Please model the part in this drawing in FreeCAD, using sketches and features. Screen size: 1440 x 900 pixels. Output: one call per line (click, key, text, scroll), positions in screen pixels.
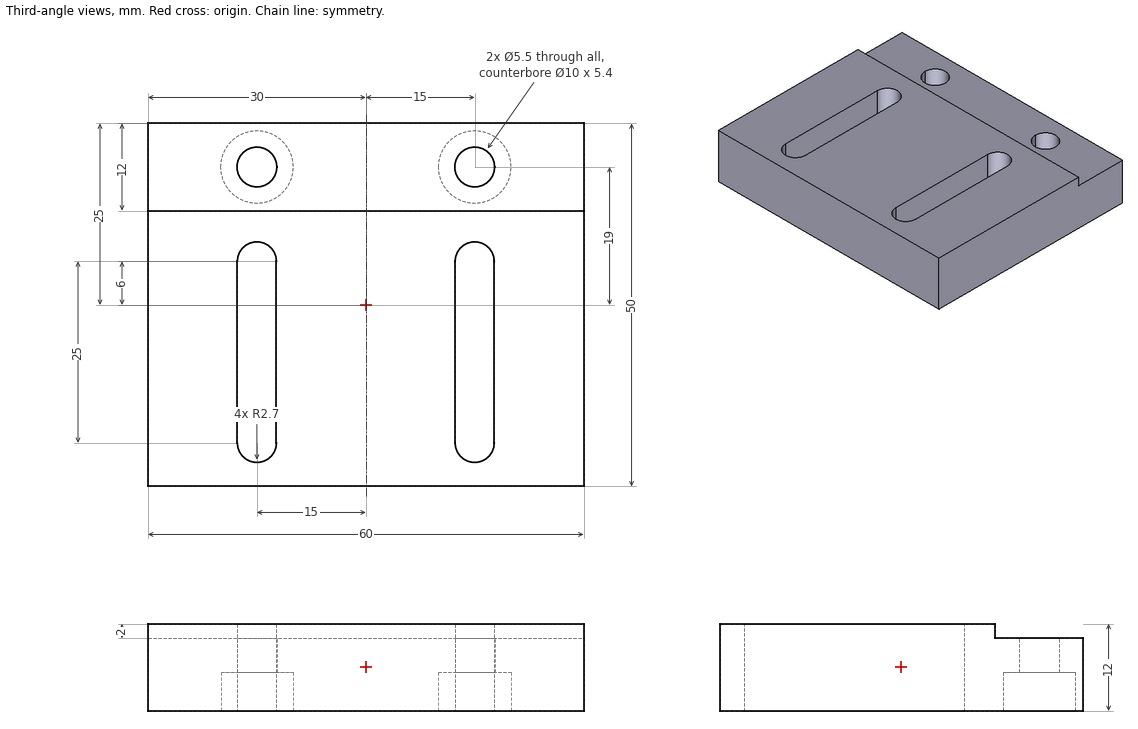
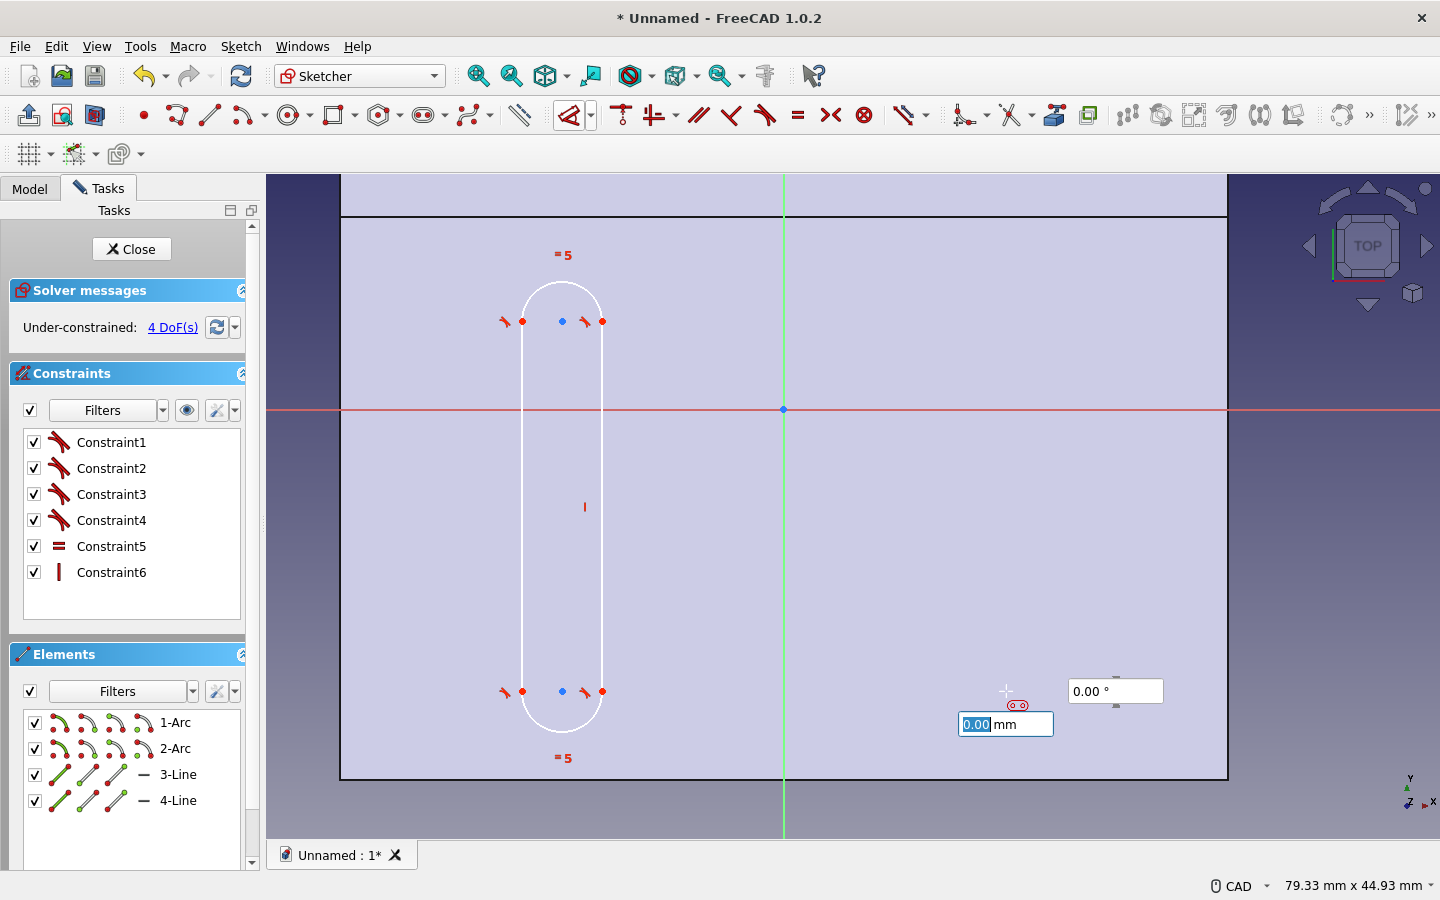
click(1006, 321)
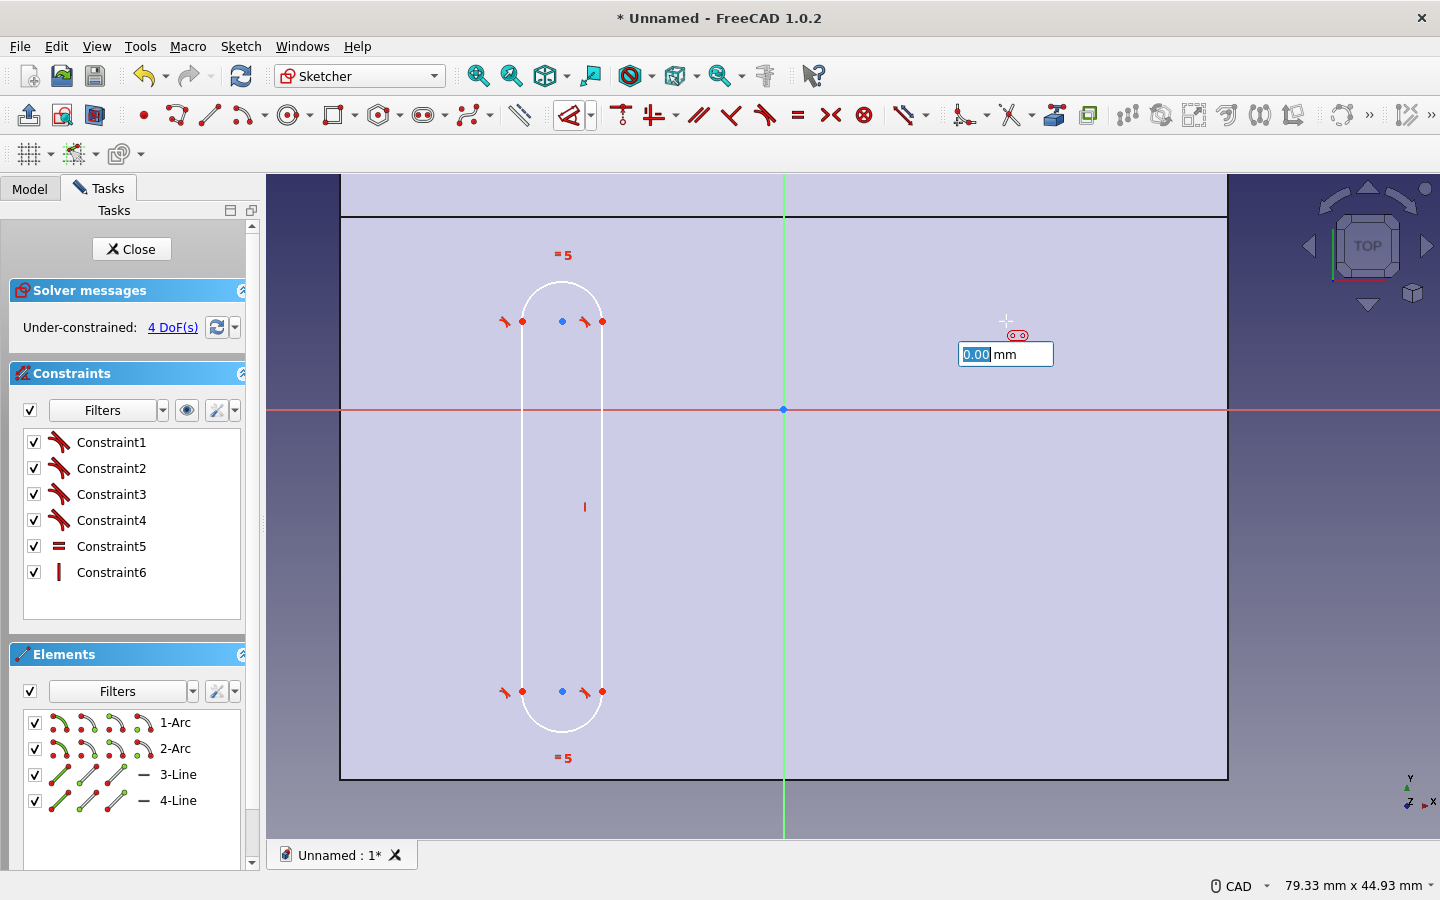
click(966, 506)
key(Escape)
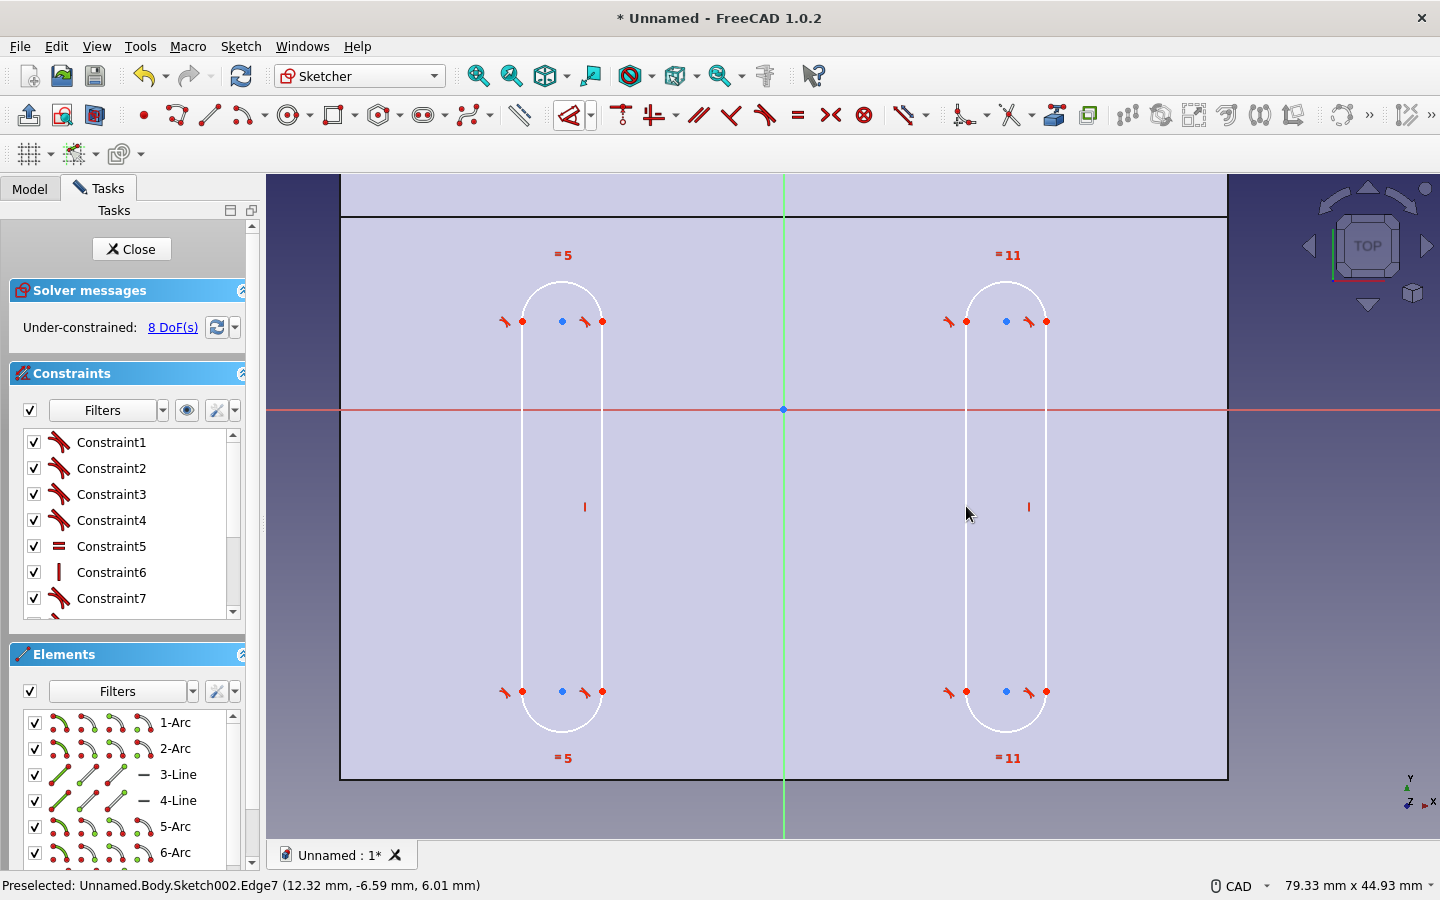
click(538, 724)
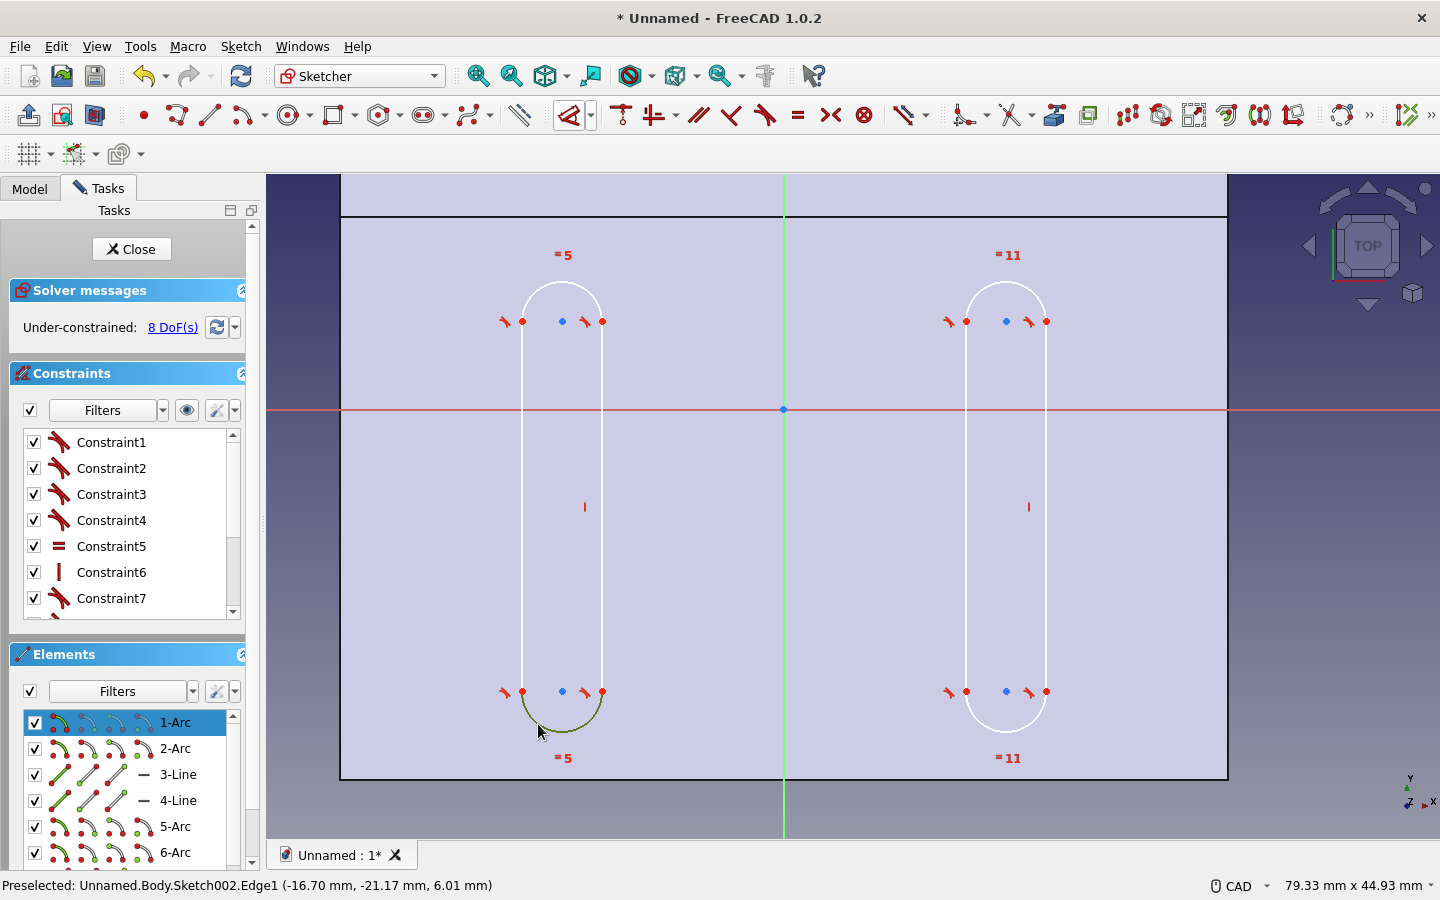
click(982, 724)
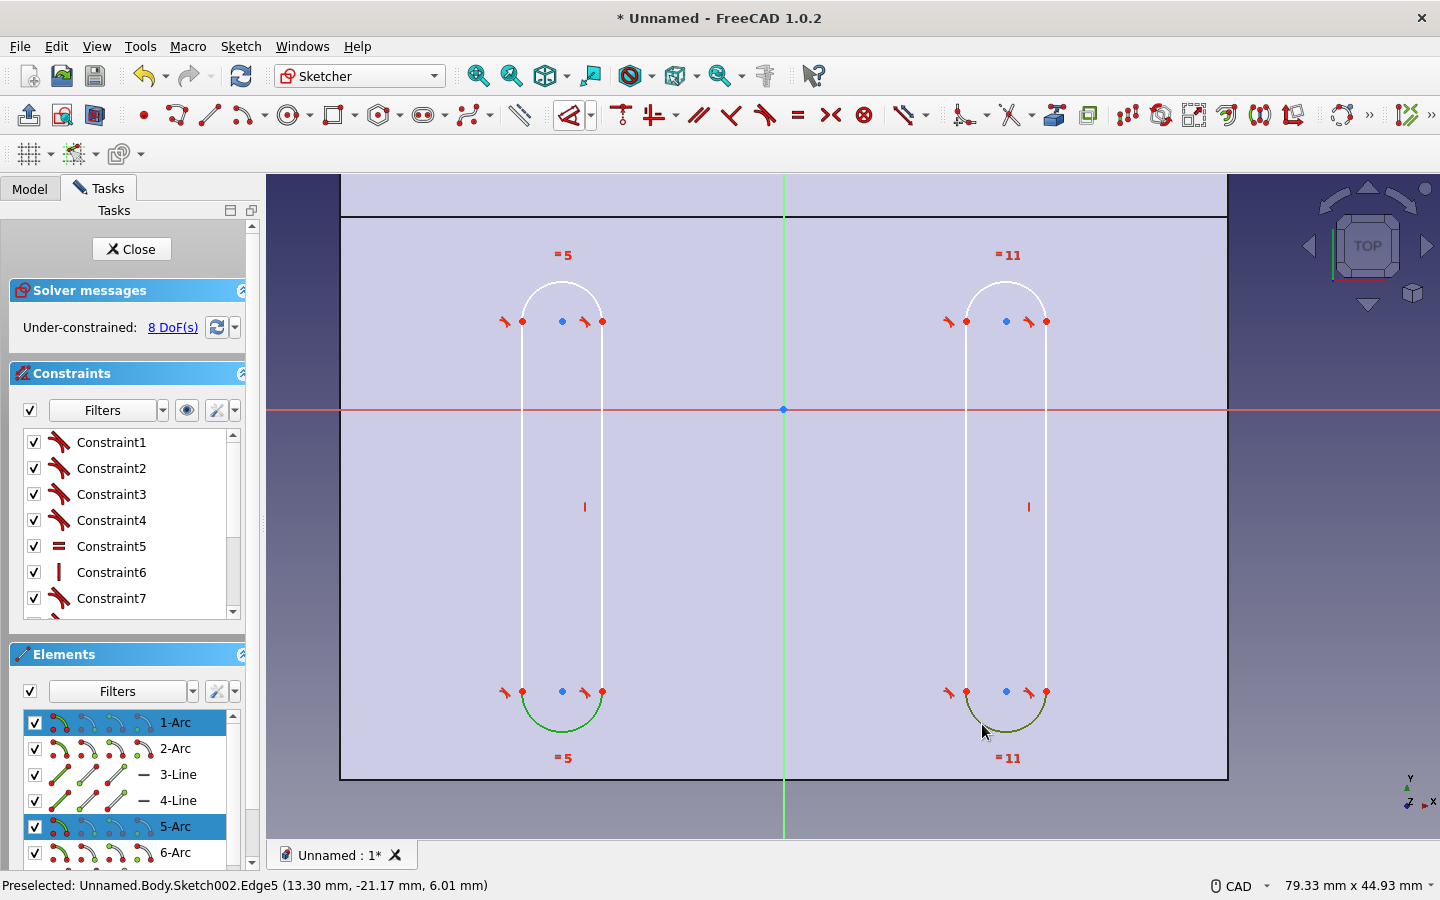
key(e)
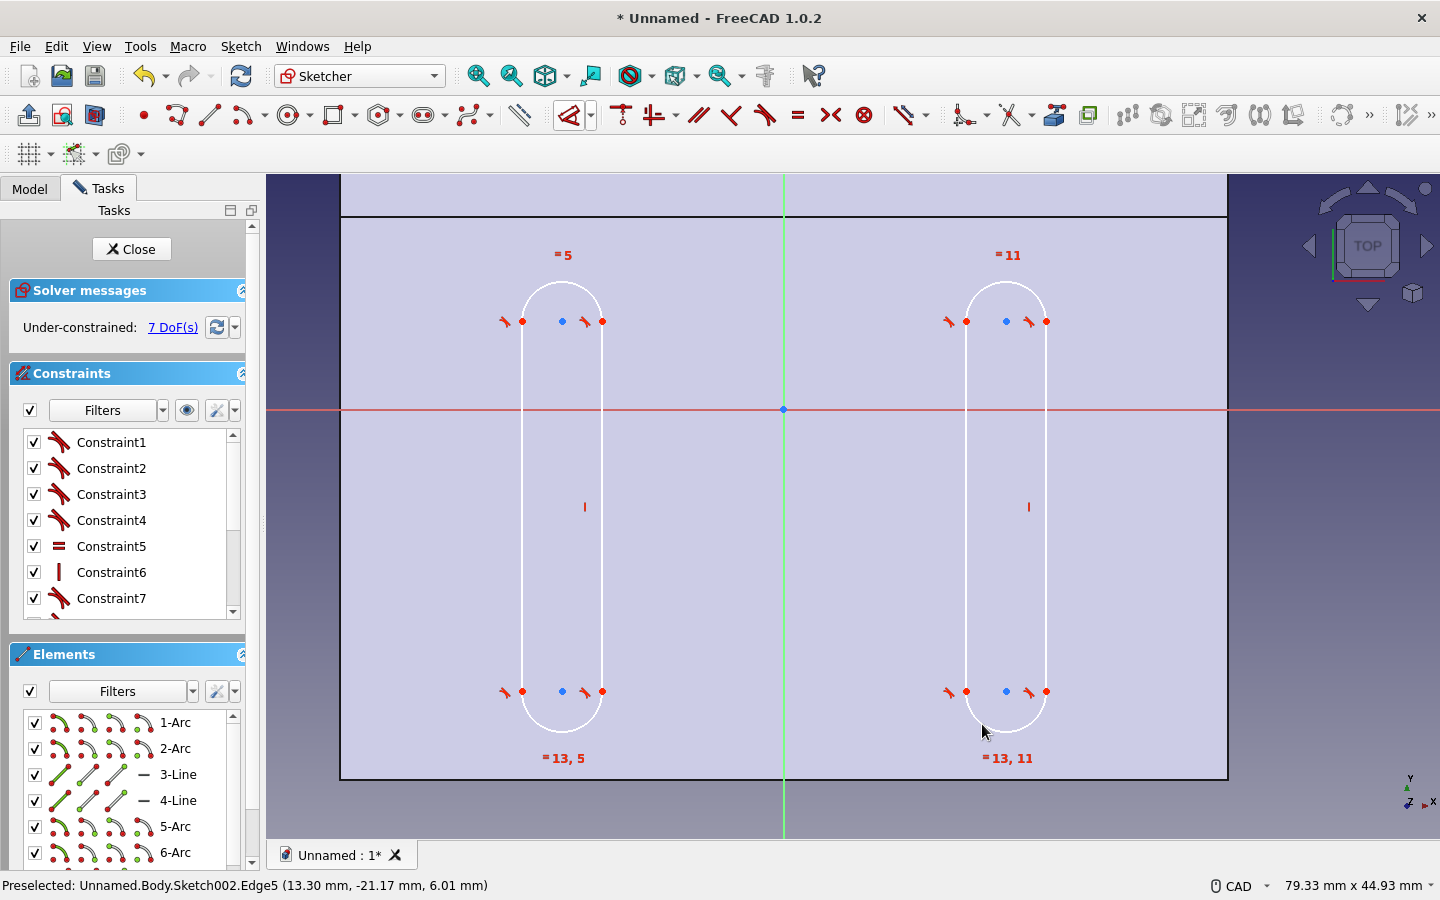
click(562, 692)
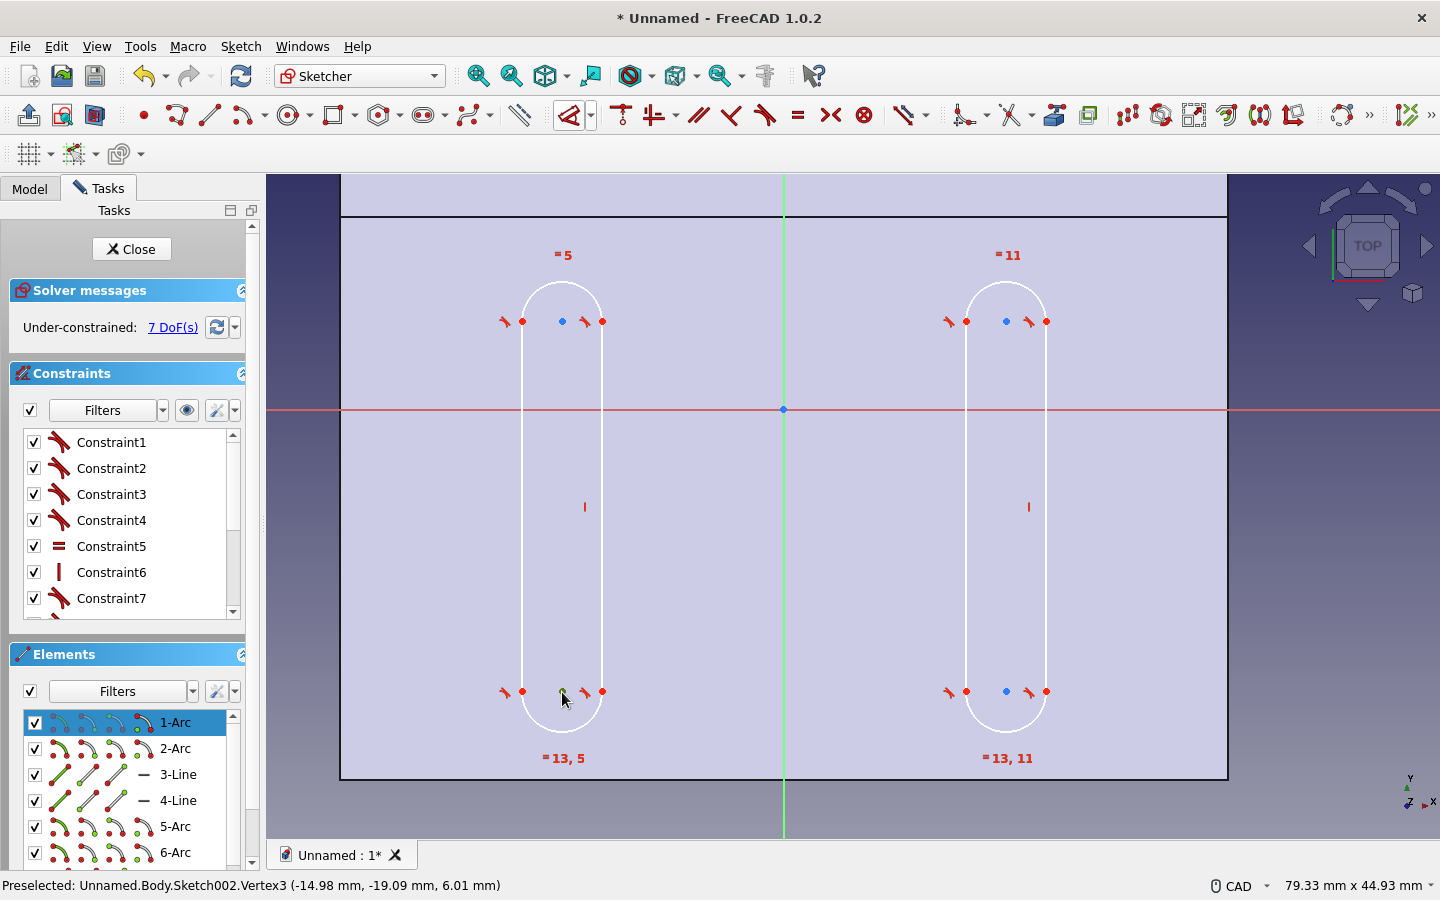
click(1006, 692)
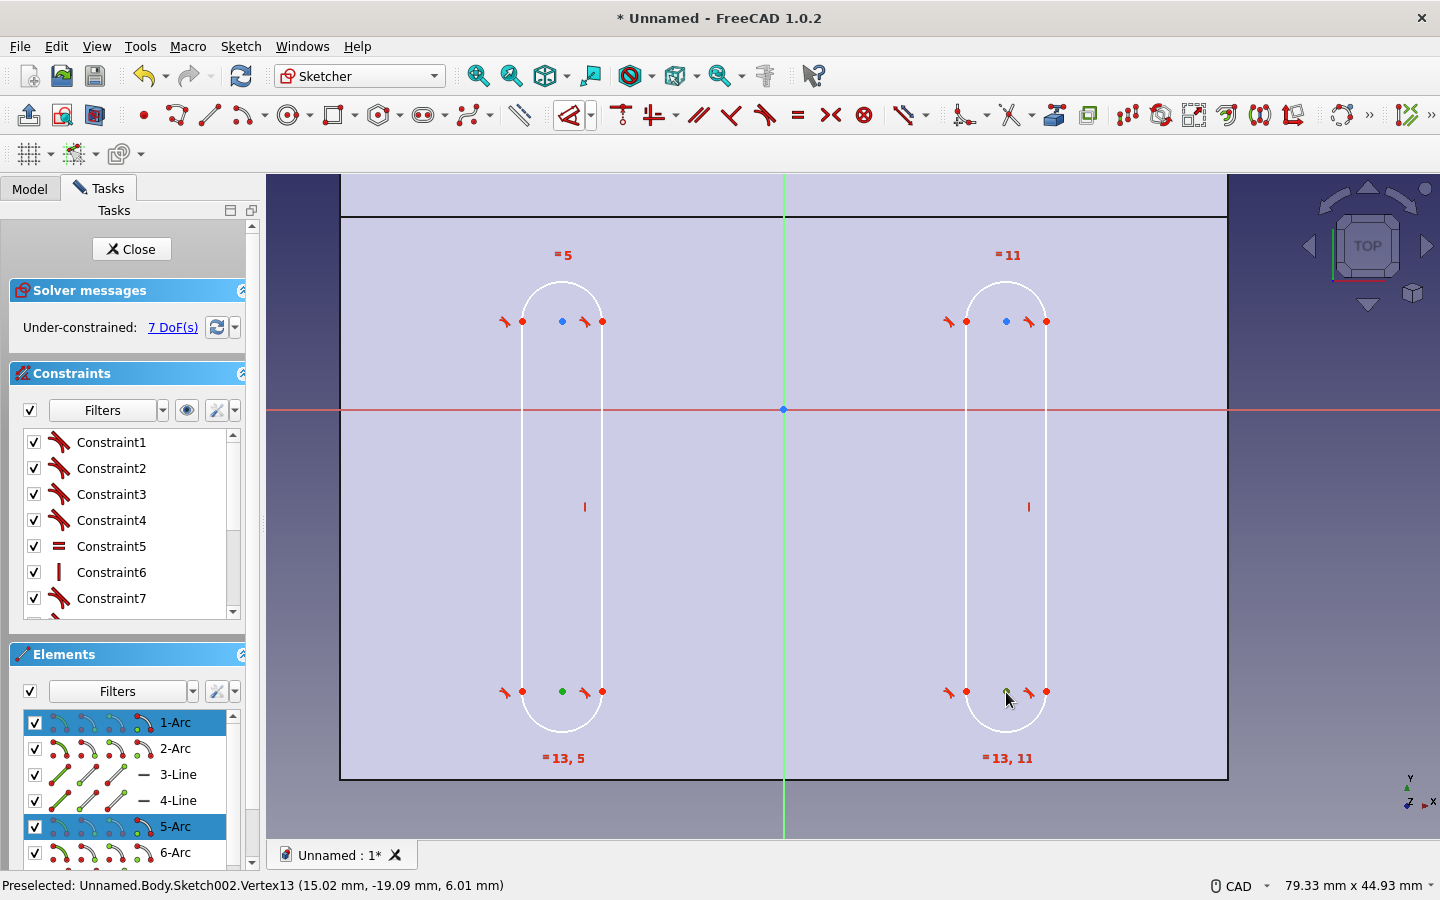
click(784, 768)